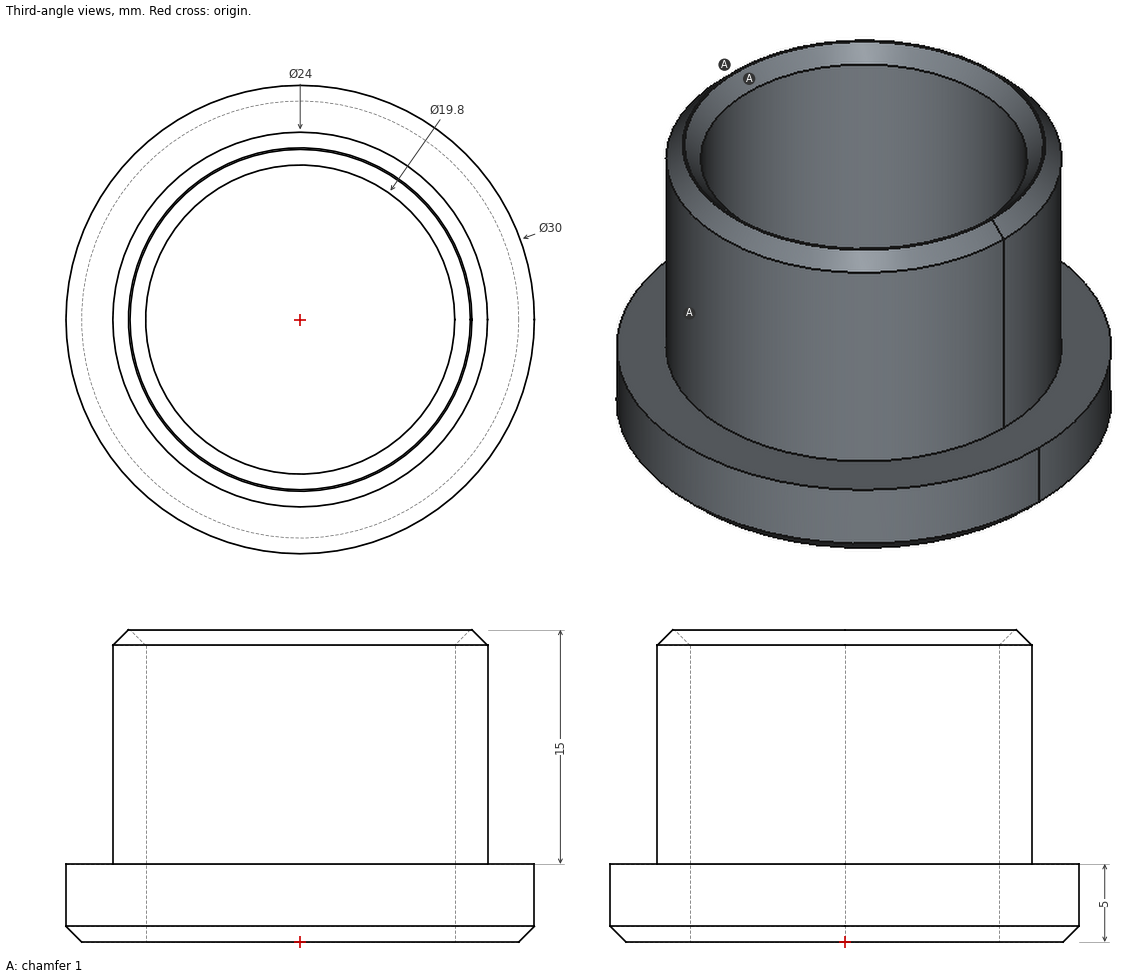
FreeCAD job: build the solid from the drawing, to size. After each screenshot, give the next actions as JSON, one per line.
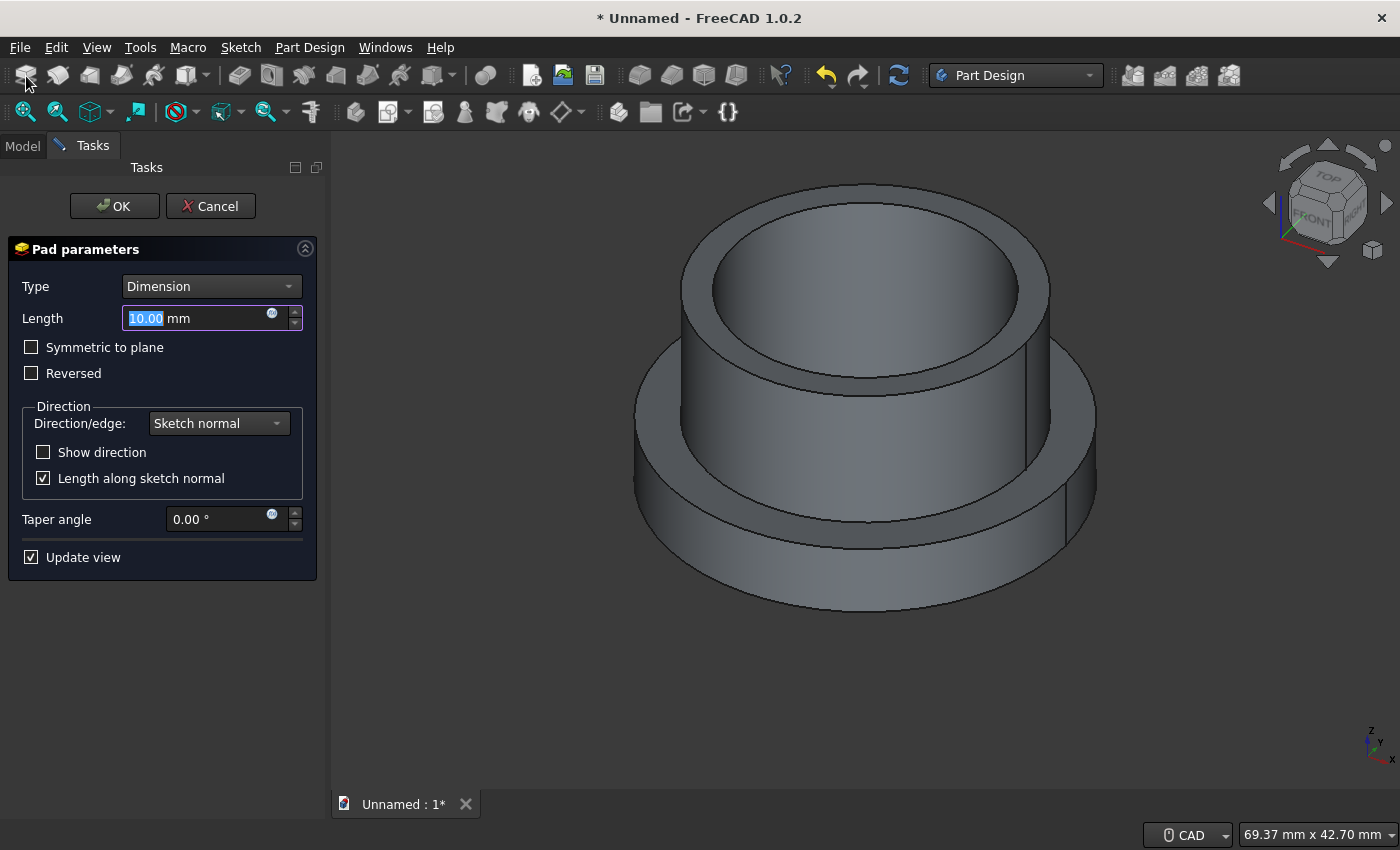
{"action": "type", "text": "15"}
{"action": "key", "text": "Tab"}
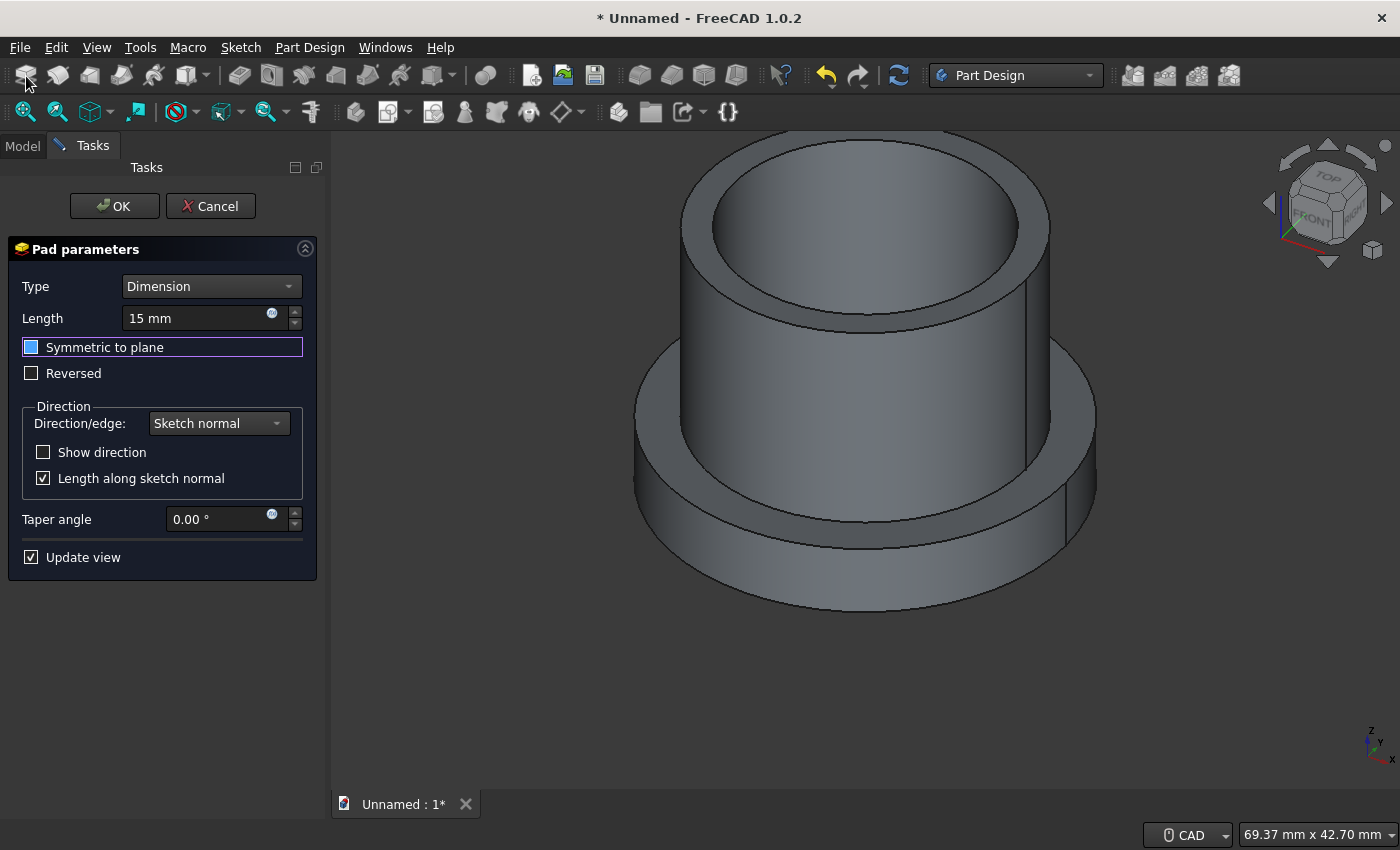
{"action": "left_click", "coordinate": [115, 206]}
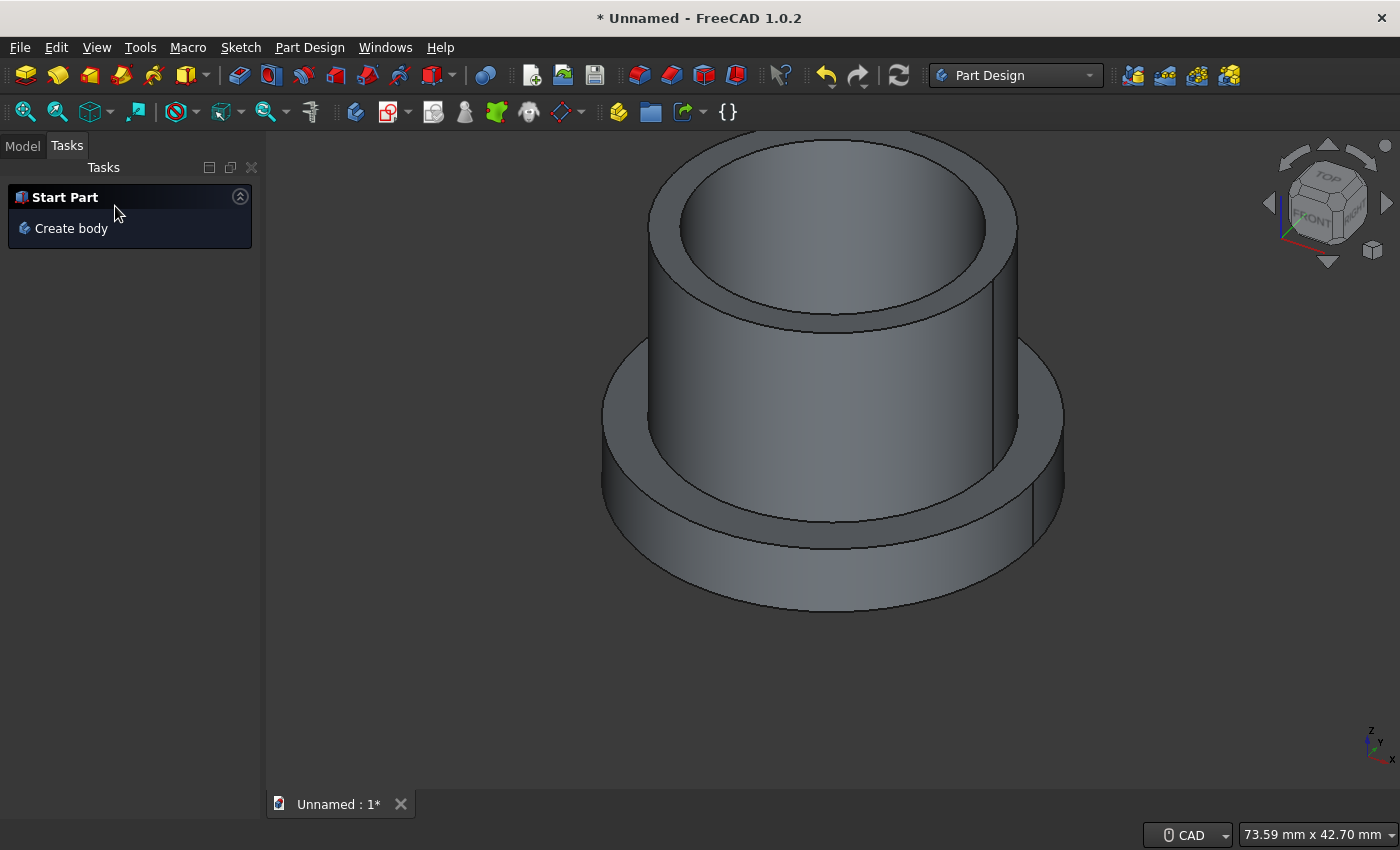
{"action": "left_click", "coordinate": [26, 112]}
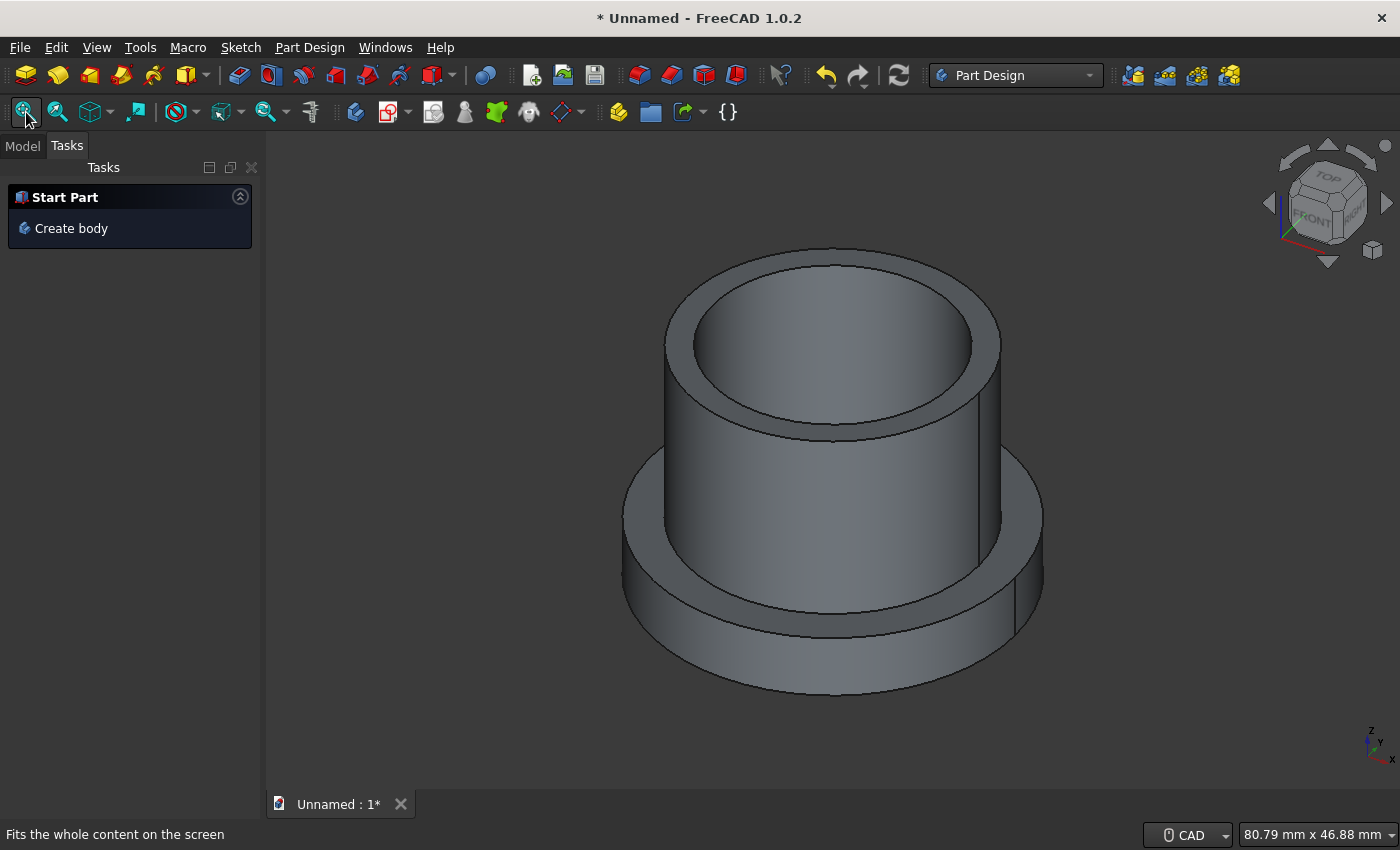
{"action": "left_click", "coordinate": [665, 354]}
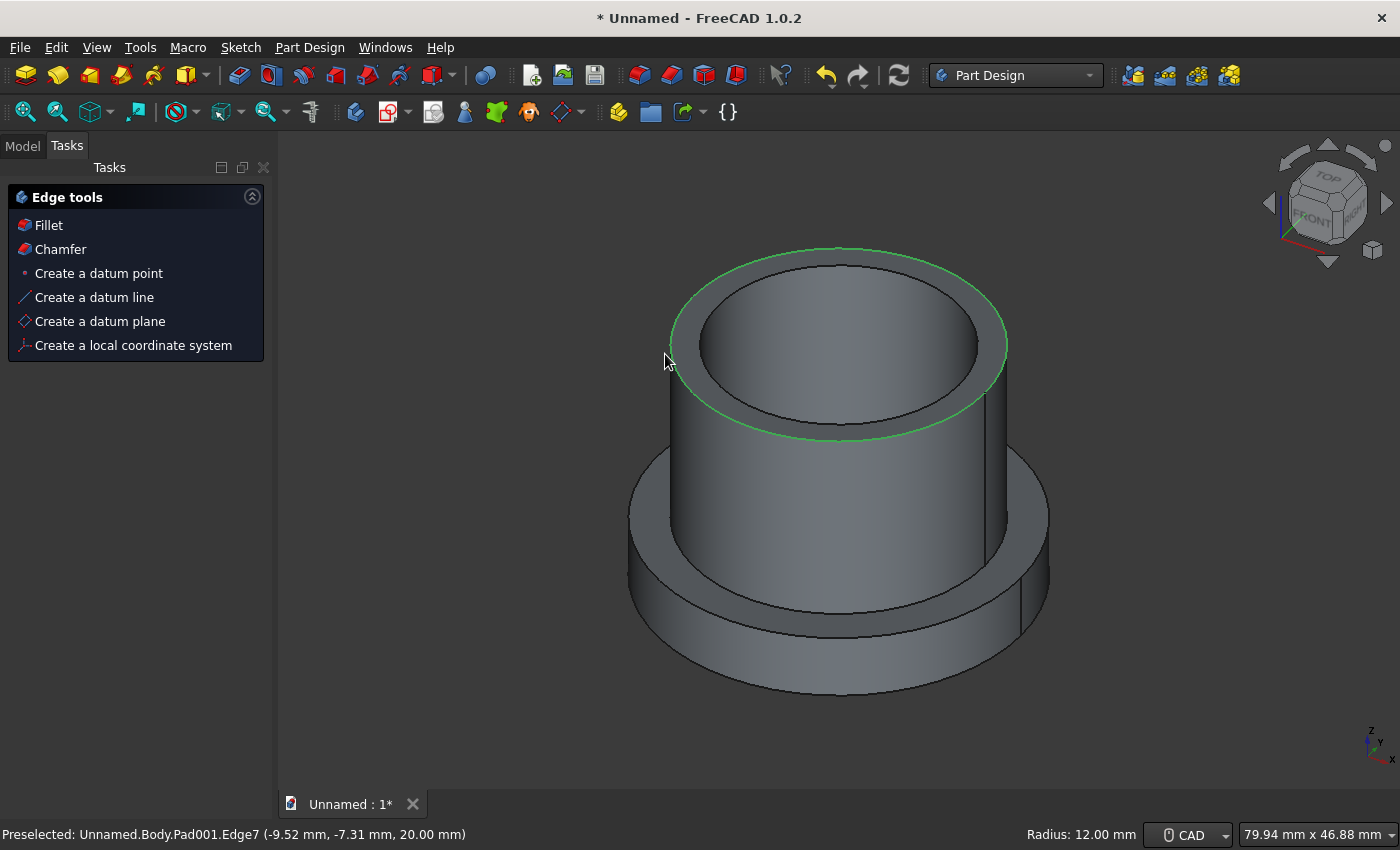
{"action": "left_click", "coordinate": [719, 304], "text": "ctrl"}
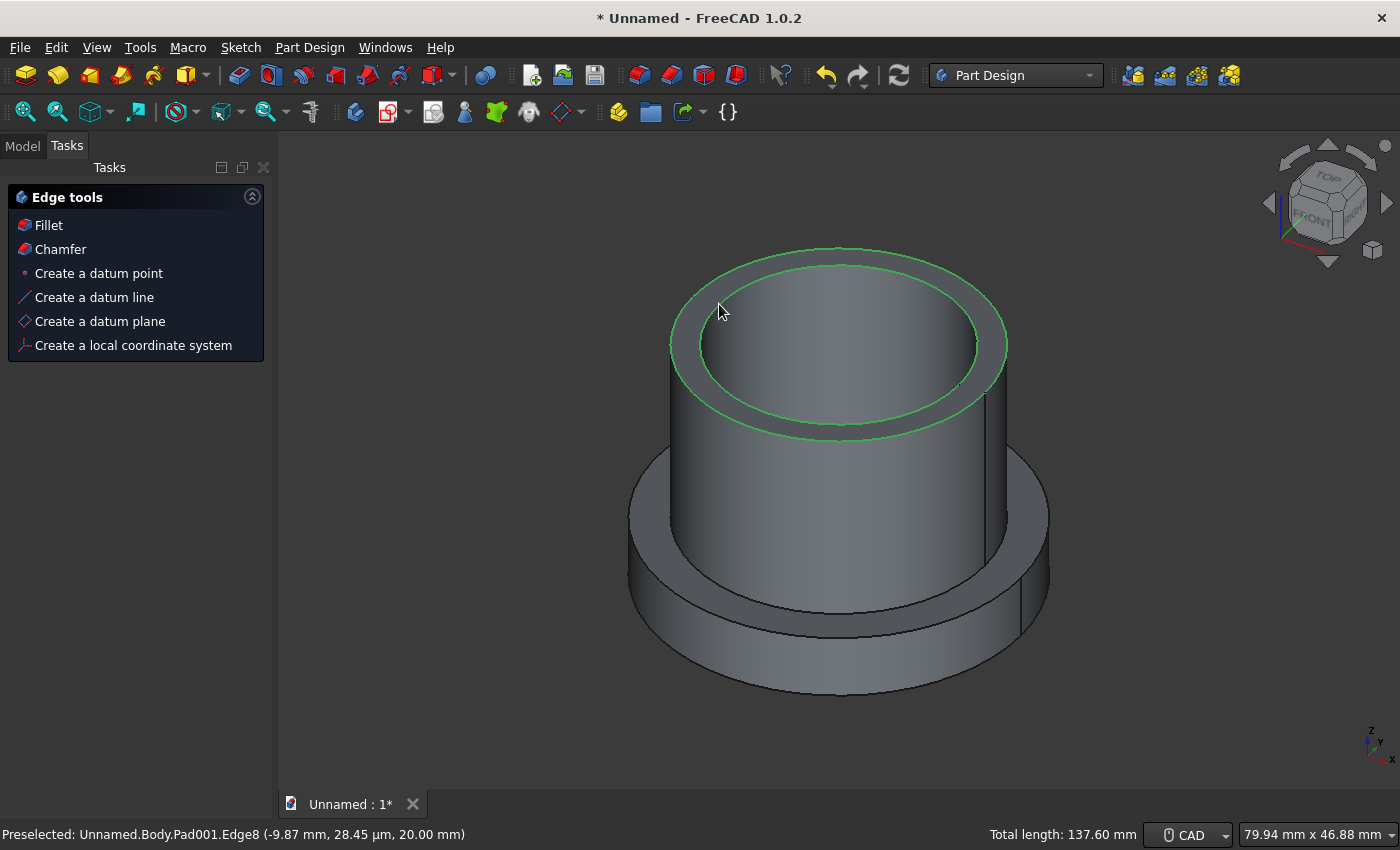
{"action": "key", "text": "0"}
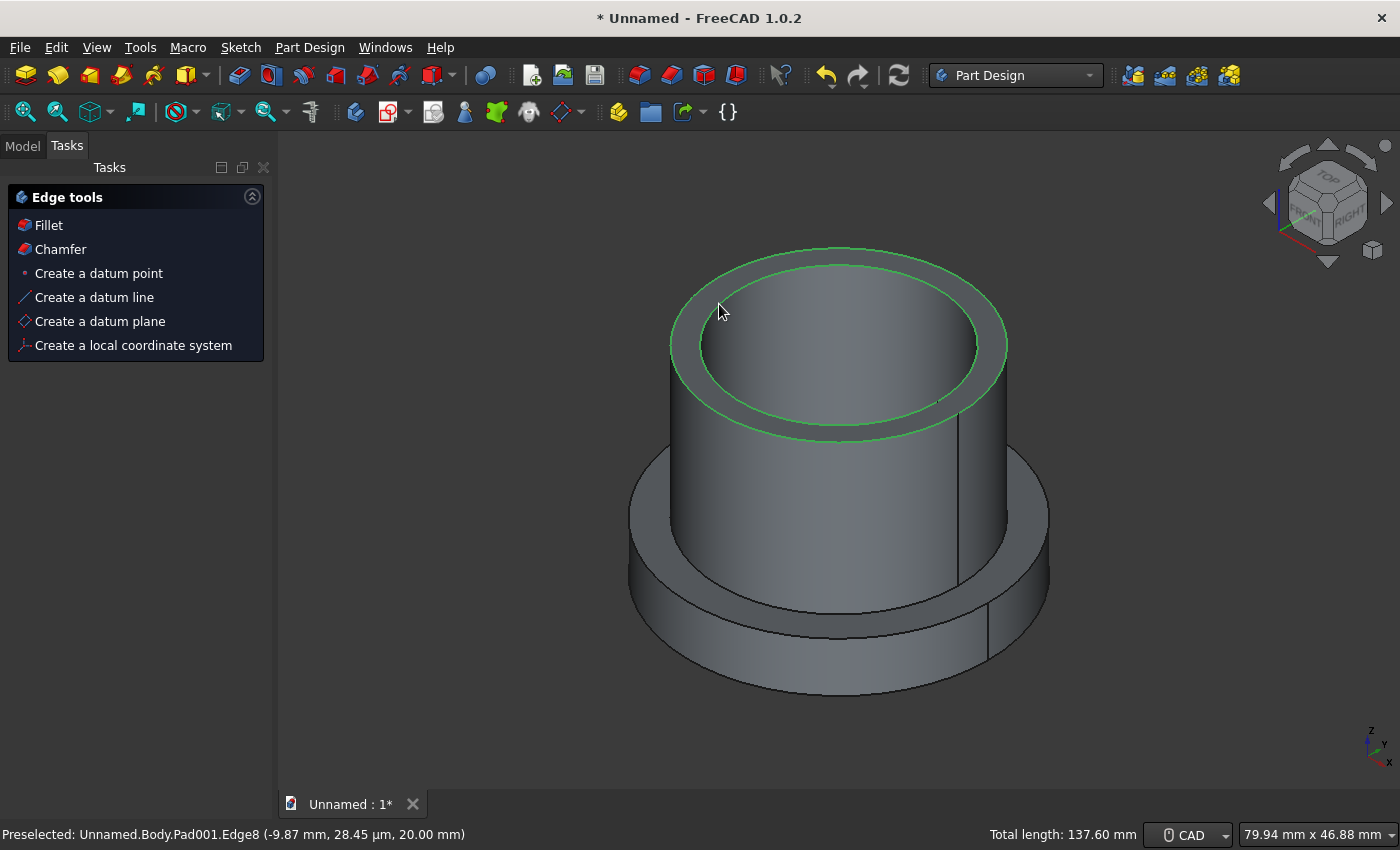
{"action": "key", "text": "2"}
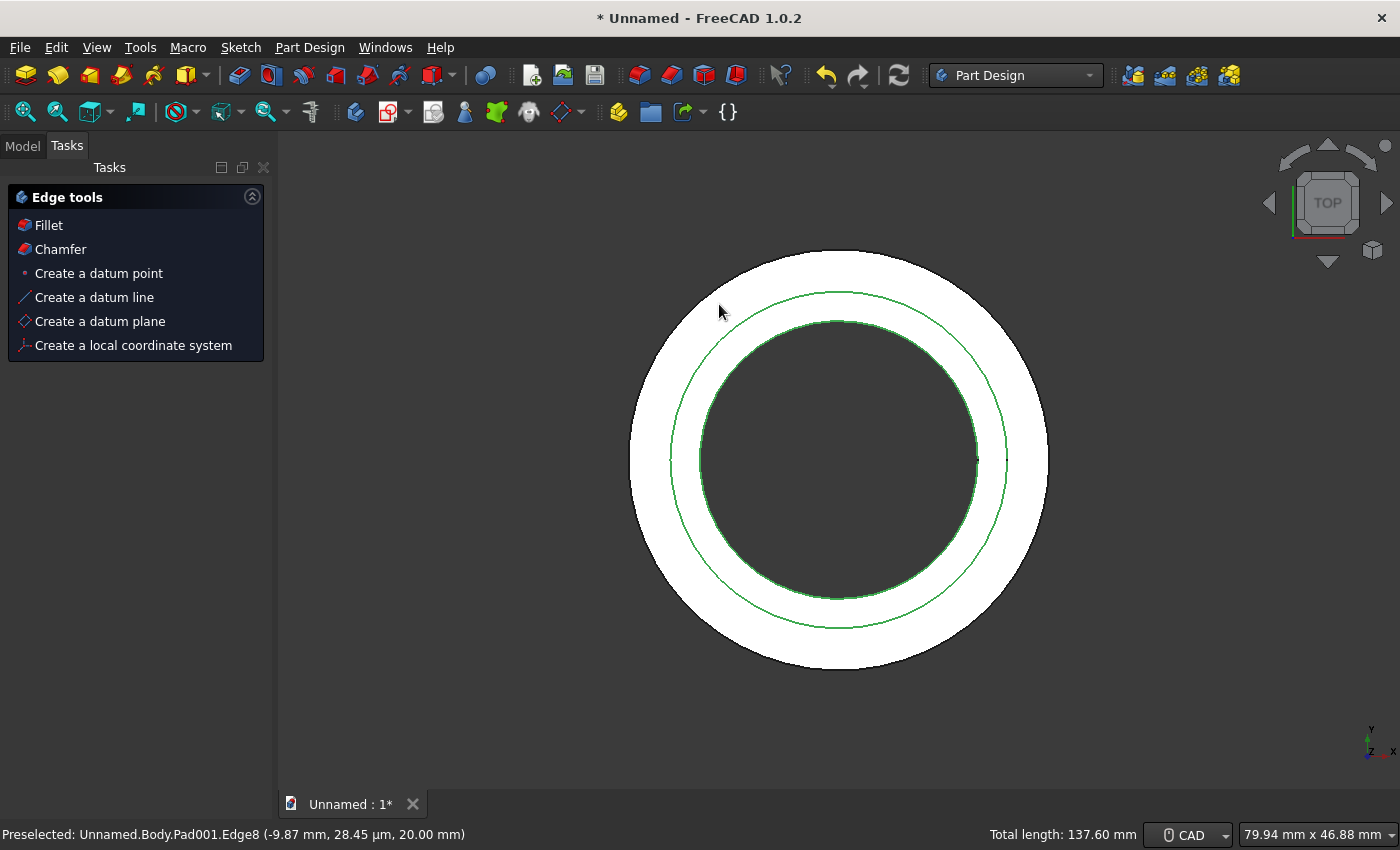
{"action": "key", "text": "1"}